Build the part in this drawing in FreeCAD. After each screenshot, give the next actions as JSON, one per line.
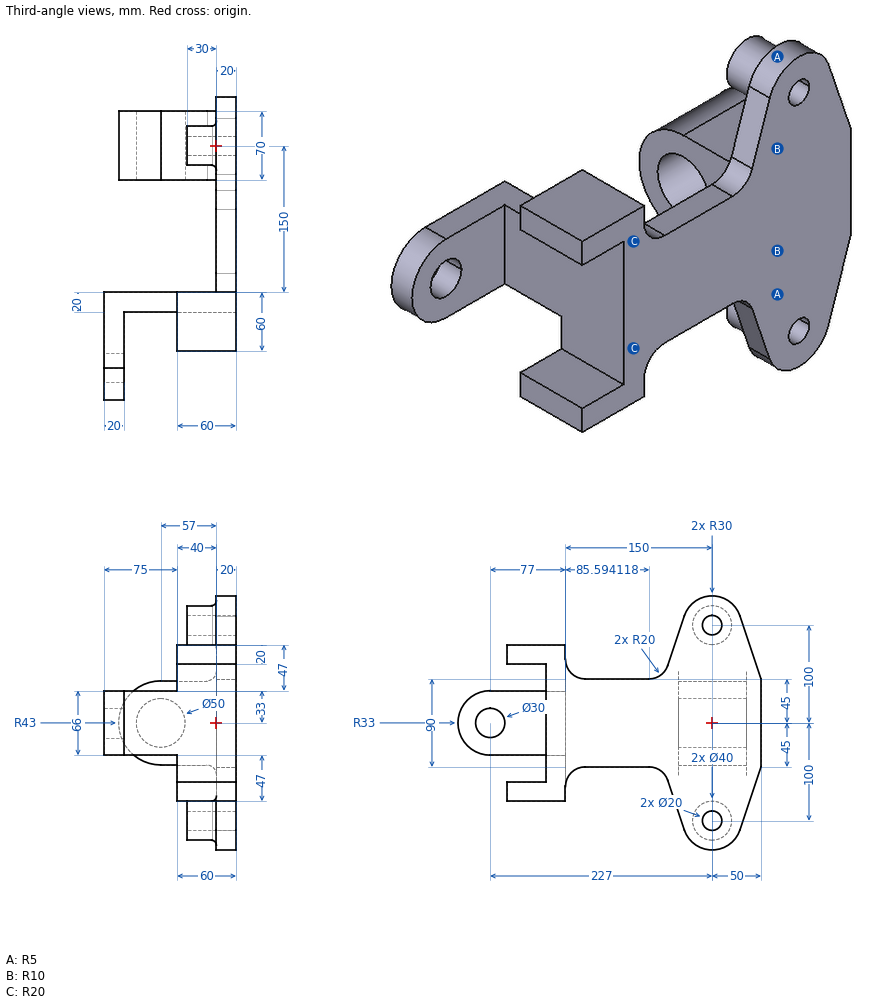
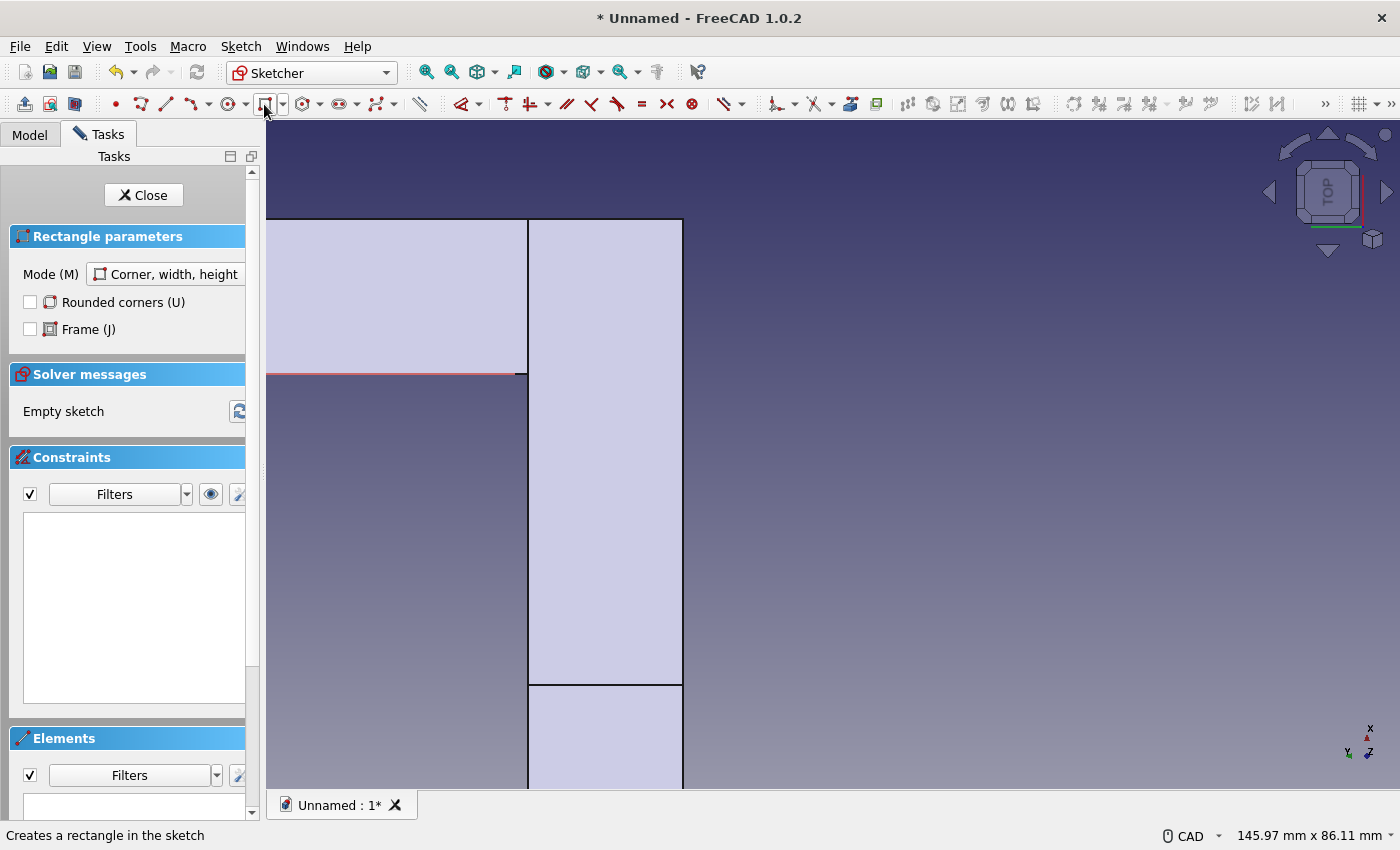
{"action": "left_click", "coordinate": [528, 219]}
{"action": "left_click", "coordinate": [994, 685]}
{"action": "key", "text": "Escape"}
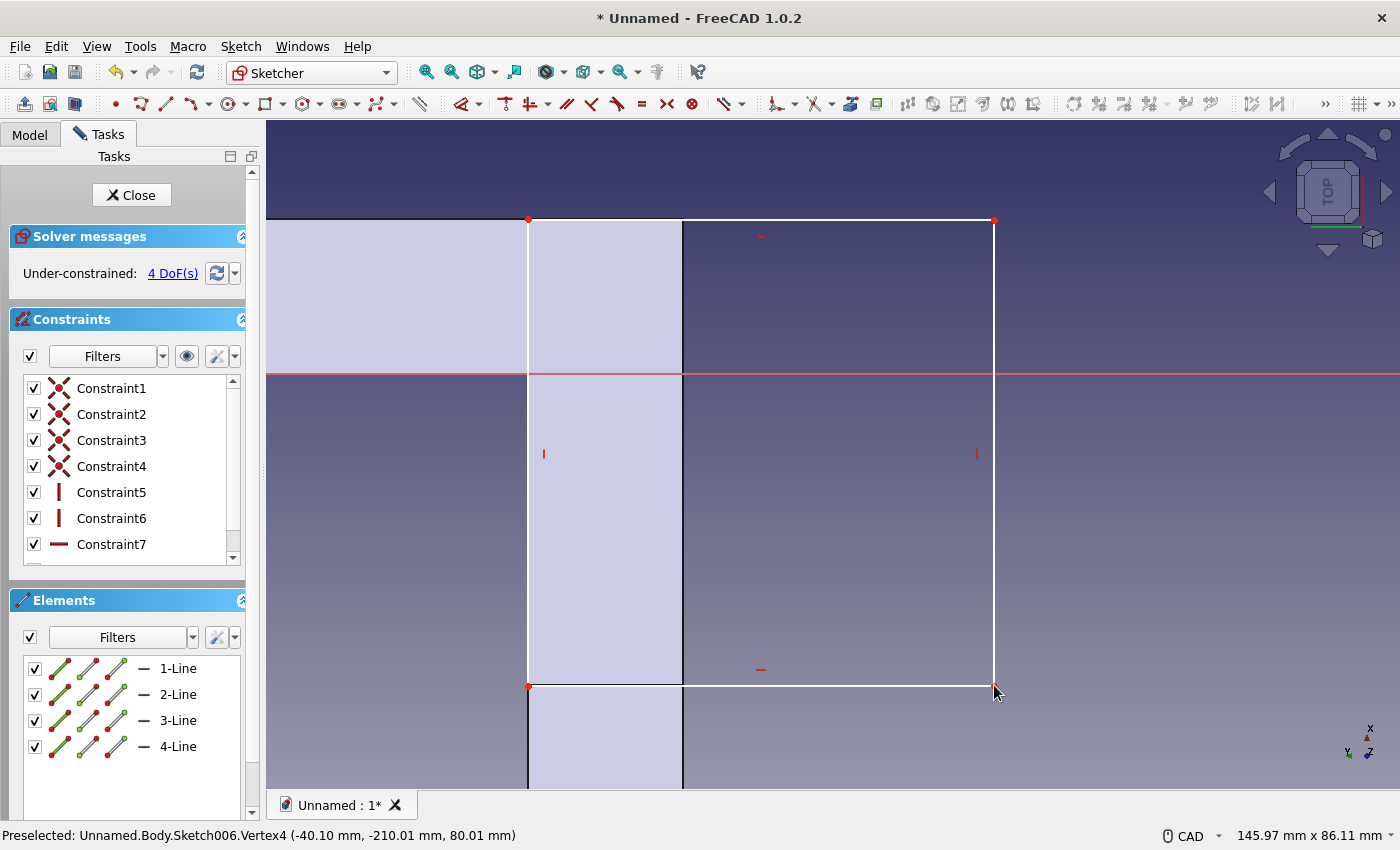
{"action": "left_click", "coordinate": [460, 104]}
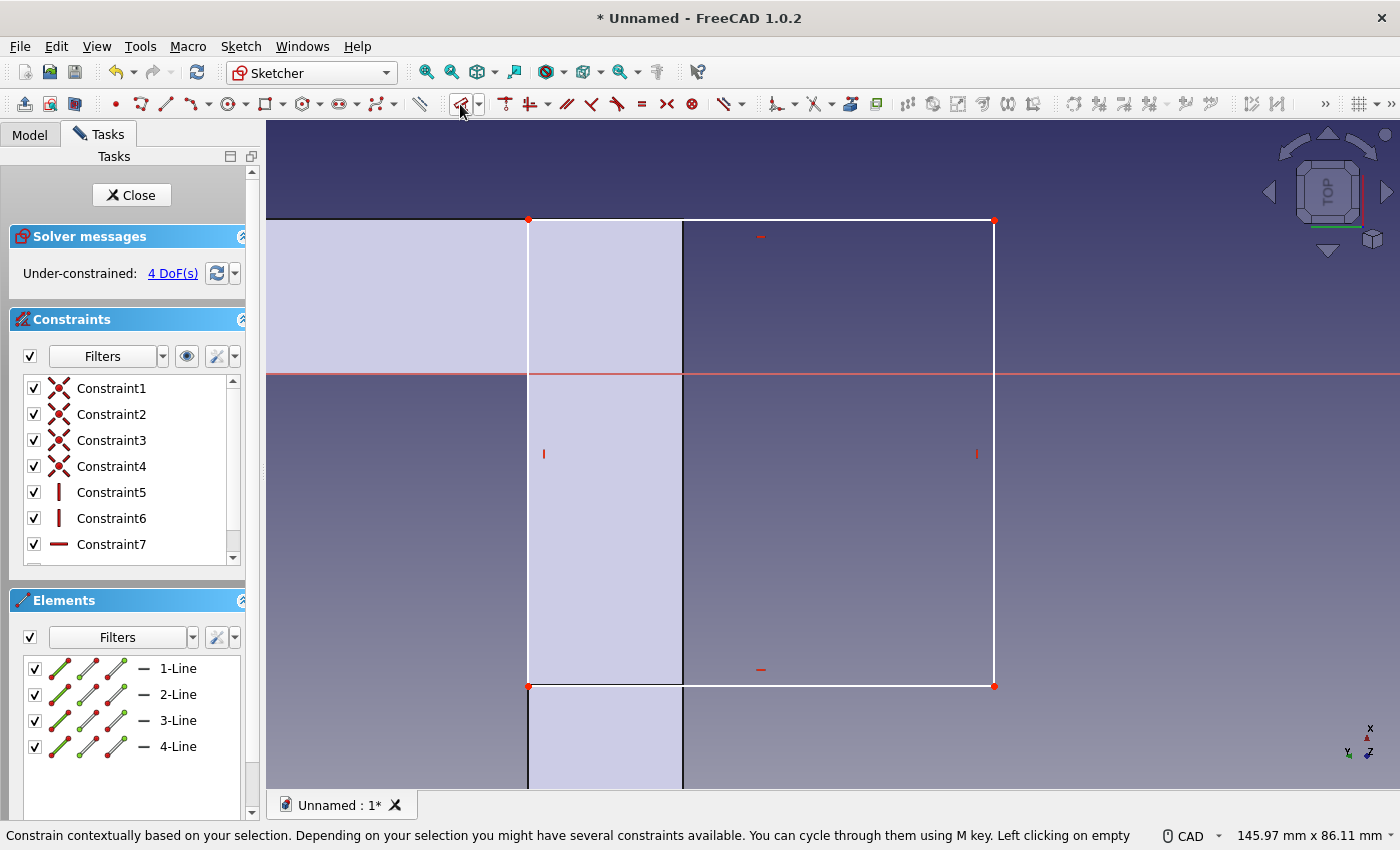
{"action": "left_click", "coordinate": [528, 360]}
{"action": "left_click", "coordinate": [494, 453]}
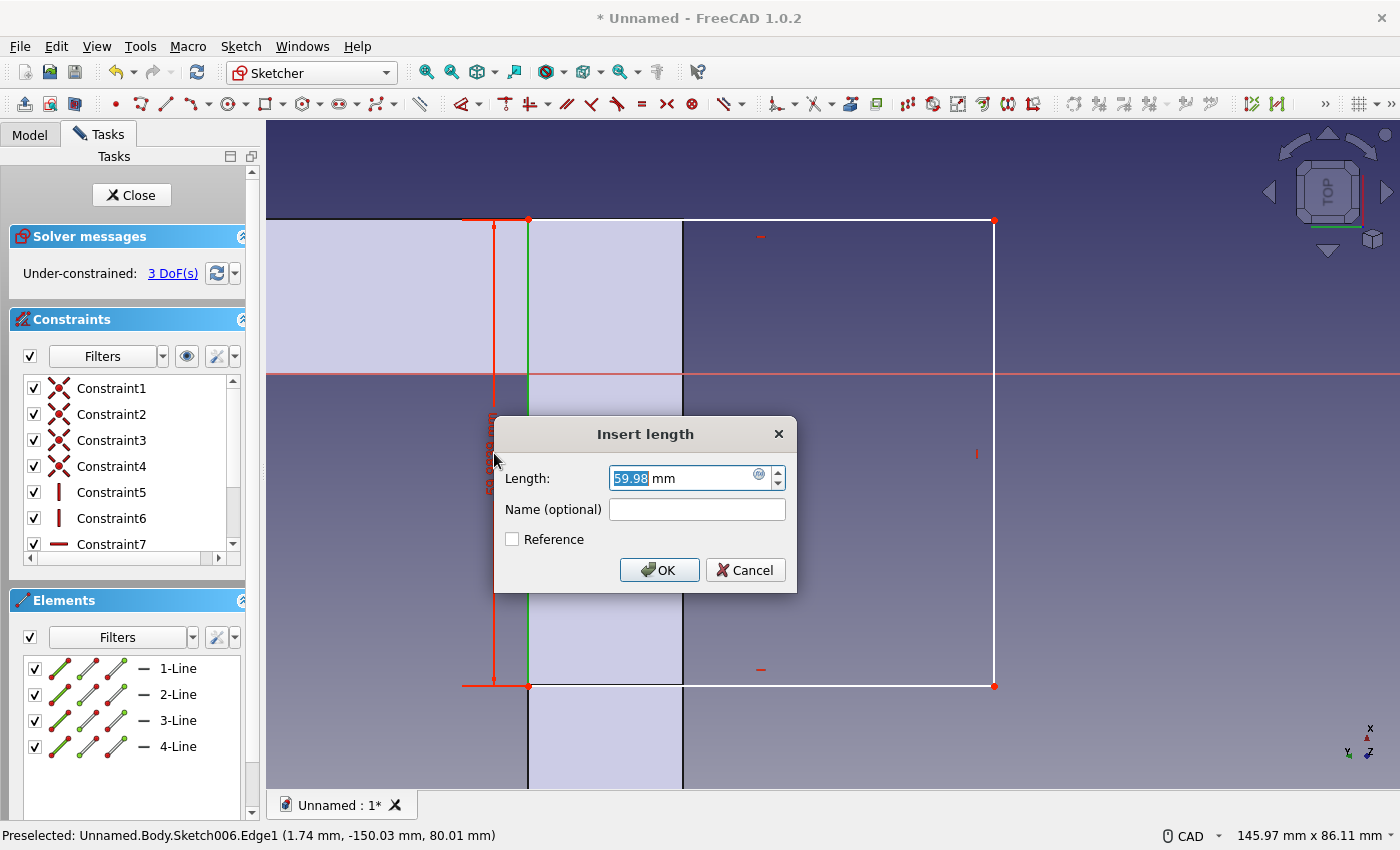
{"action": "type", "text": "60"}
{"action": "key", "text": "Return"}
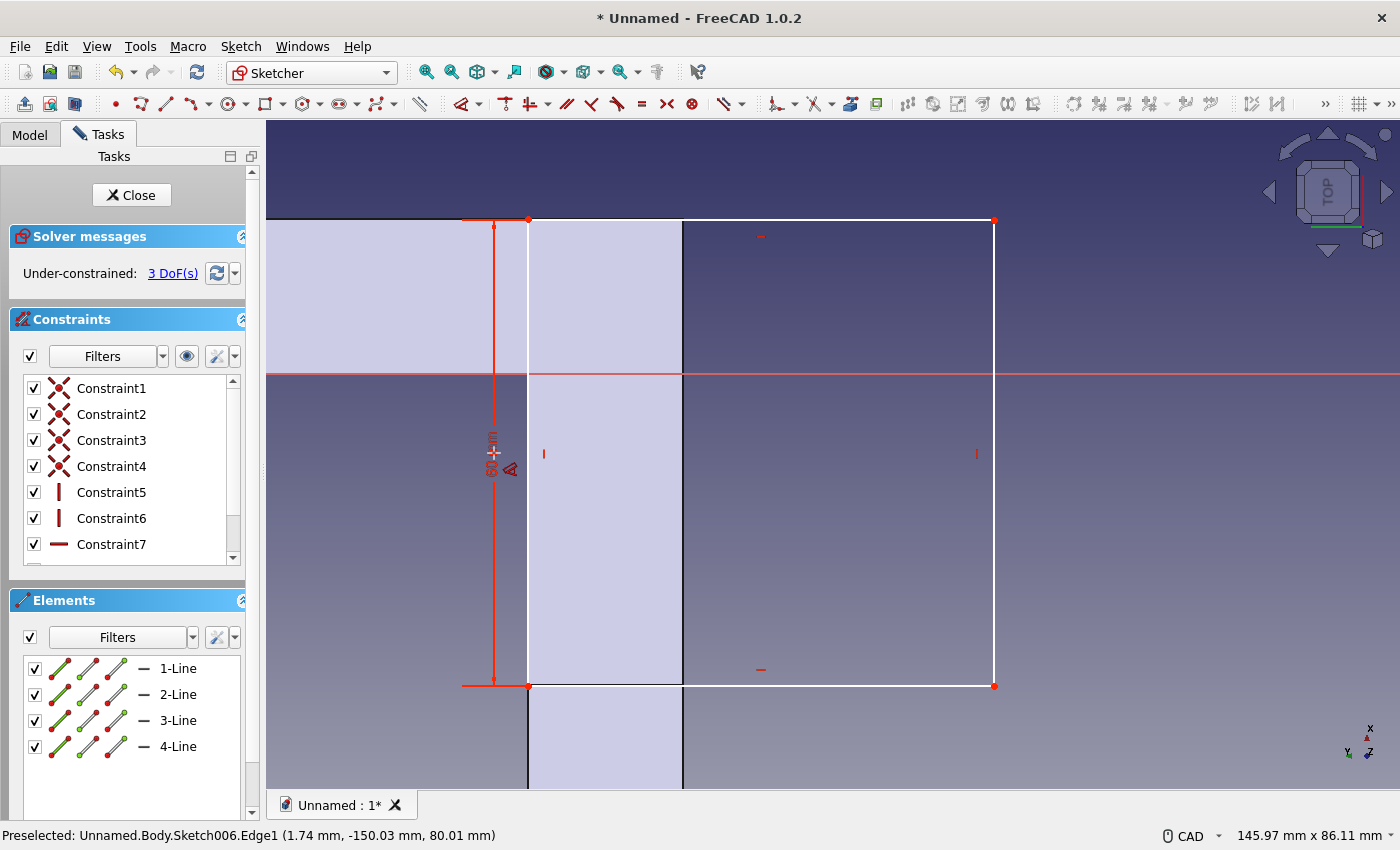
{"action": "left_click", "coordinate": [668, 686]}
{"action": "left_click", "coordinate": [761, 720]}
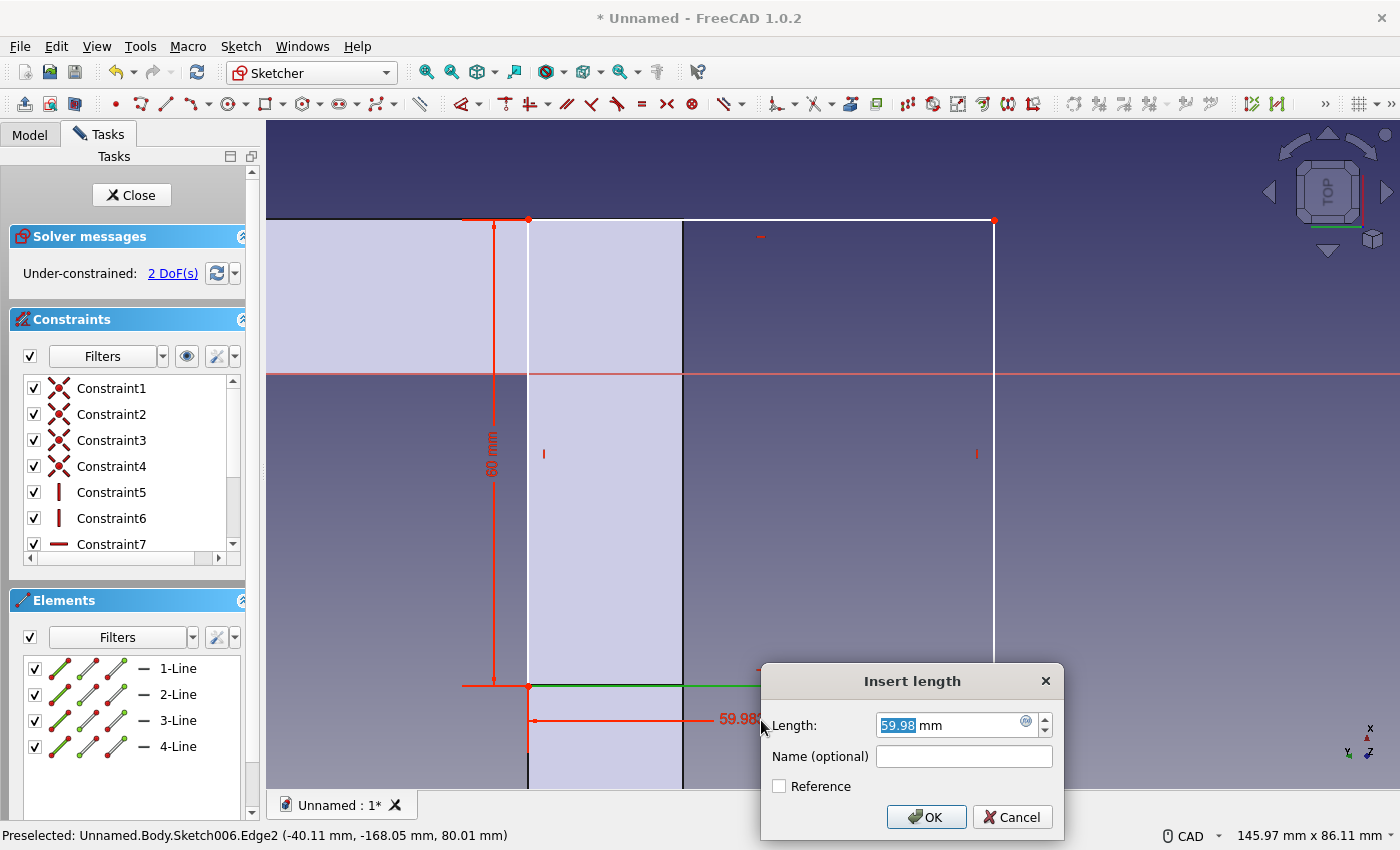
{"action": "type", "text": "60"}
{"action": "key", "text": "Return"}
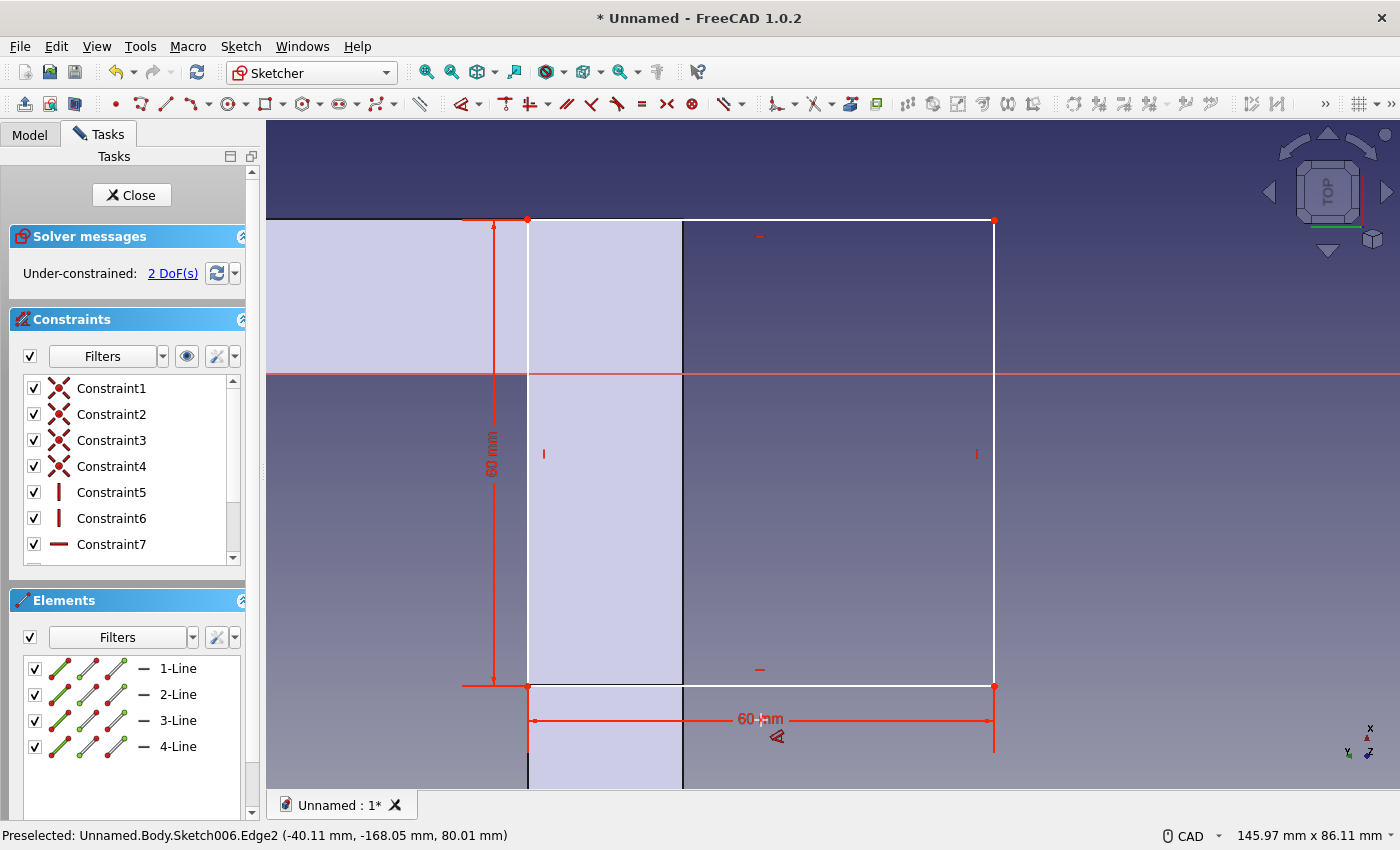
{"action": "left_click", "coordinate": [528, 220]}
{"action": "left_click", "coordinate": [562, 297]}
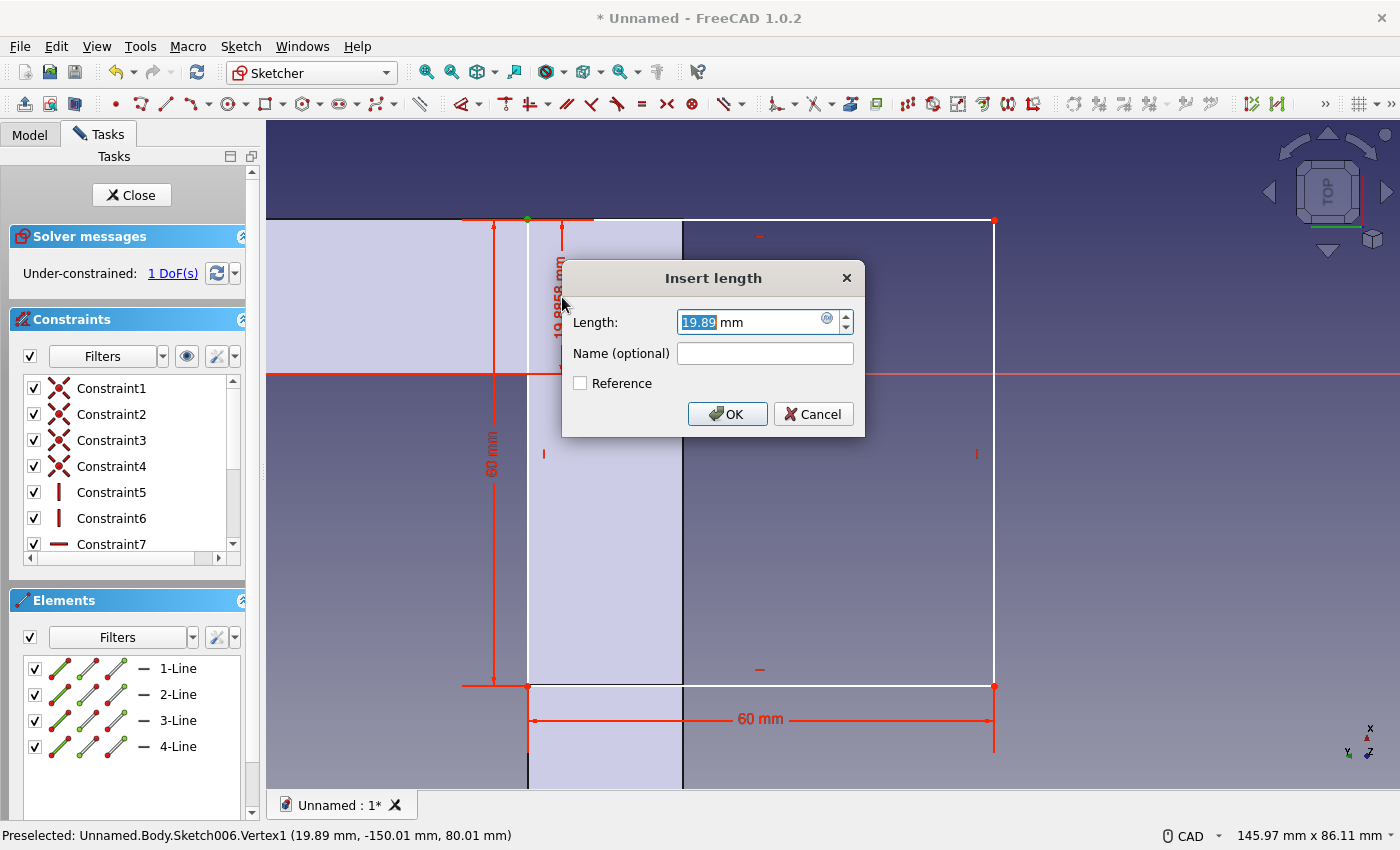
{"action": "type", "text": "20"}
{"action": "key", "text": "Return"}